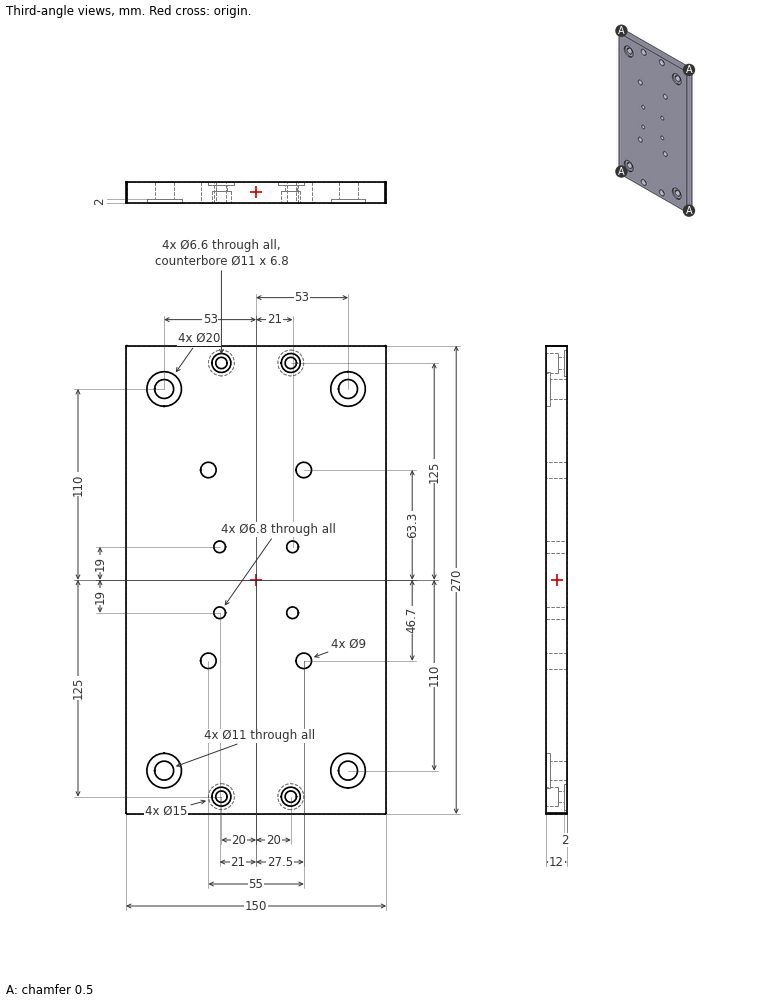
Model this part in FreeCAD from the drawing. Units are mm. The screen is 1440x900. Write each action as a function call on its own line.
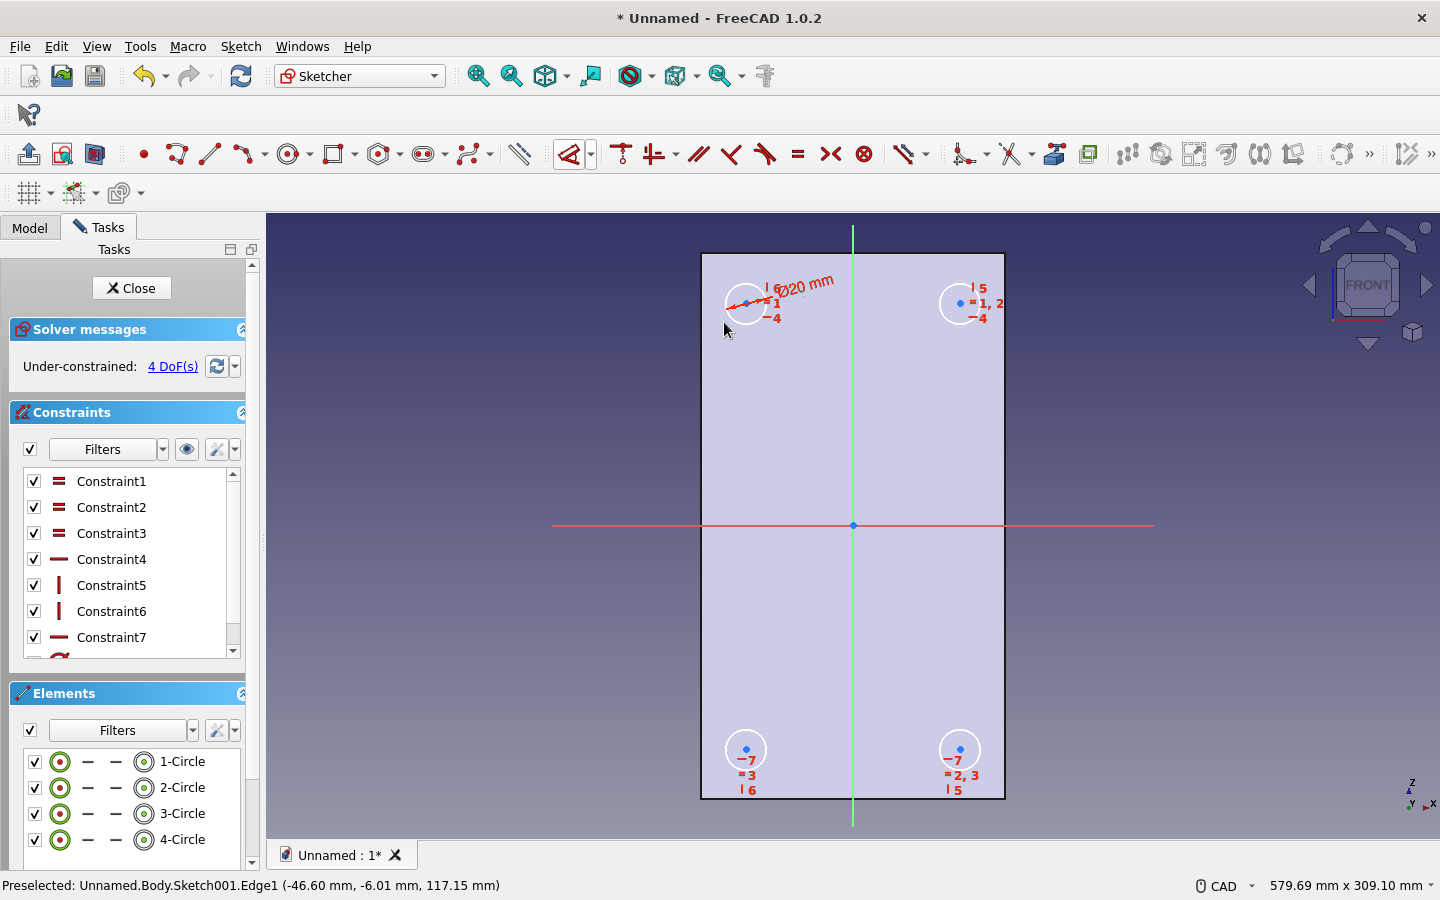
click(746, 304)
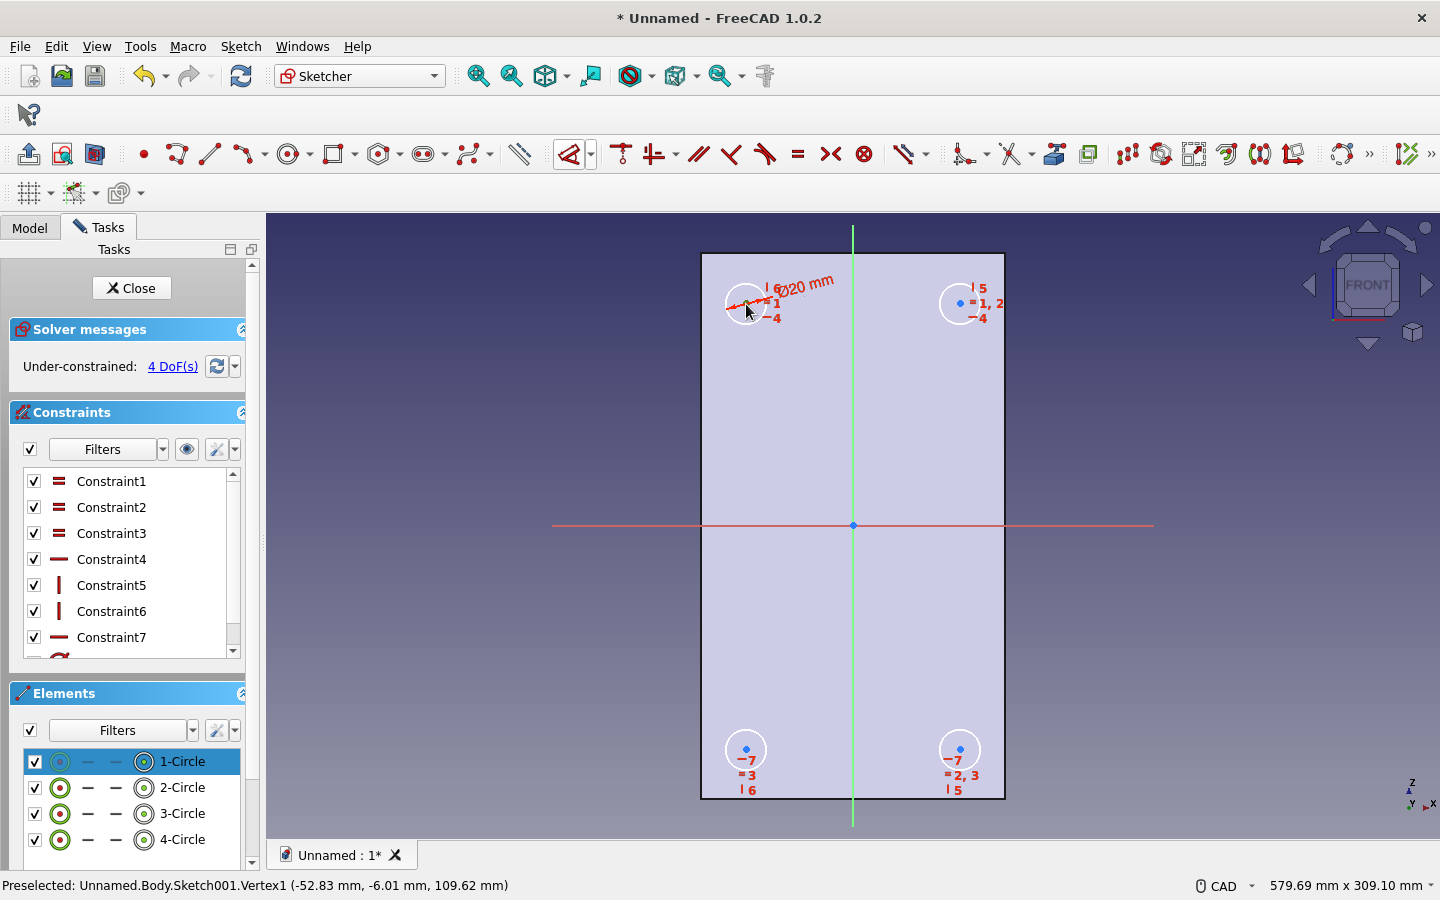
key(l)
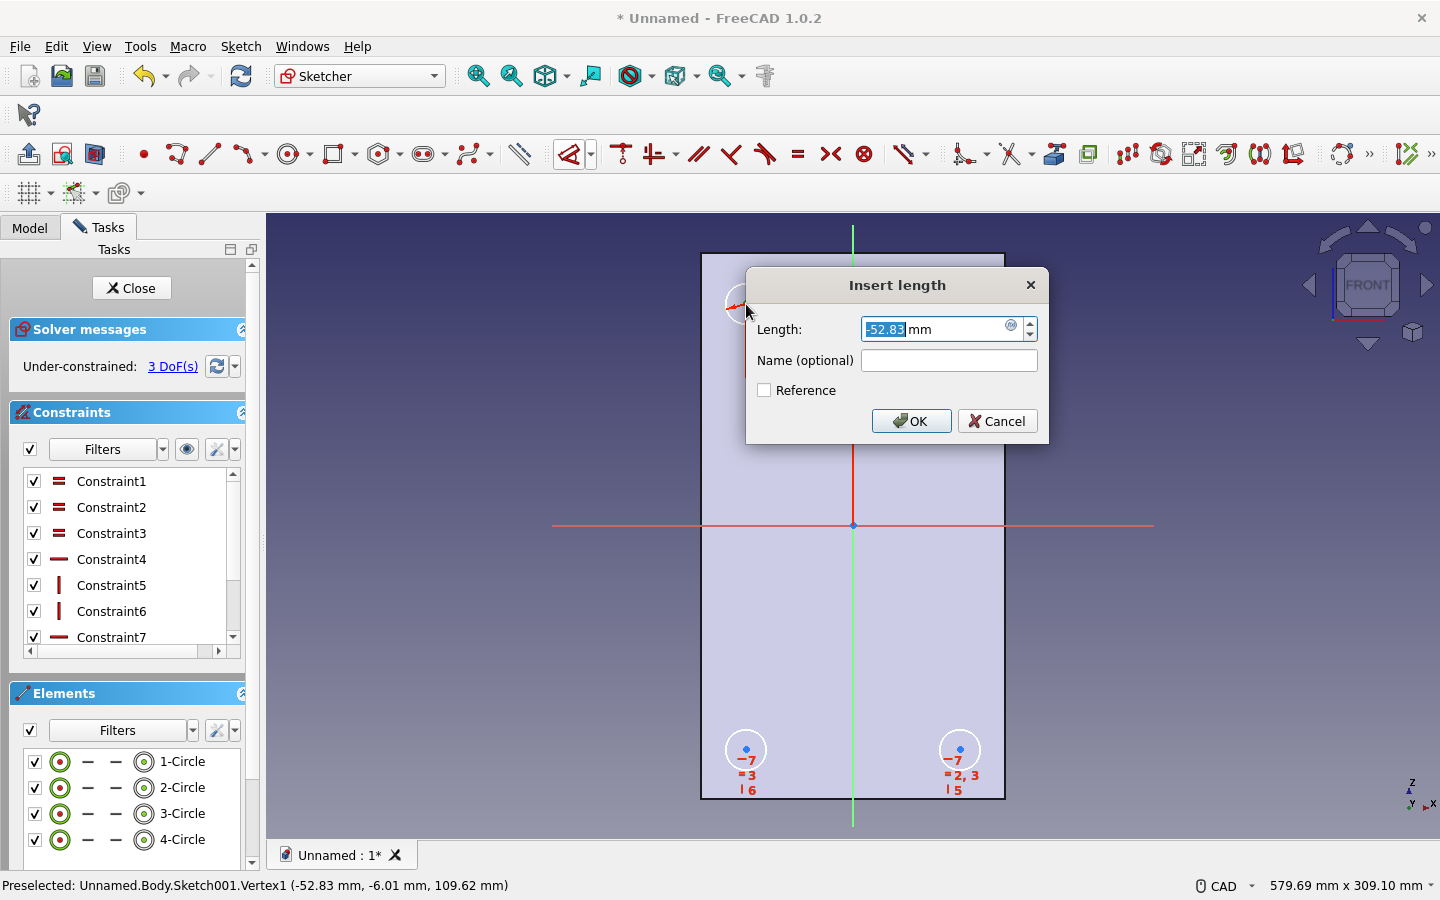
text(-53)
key(Return)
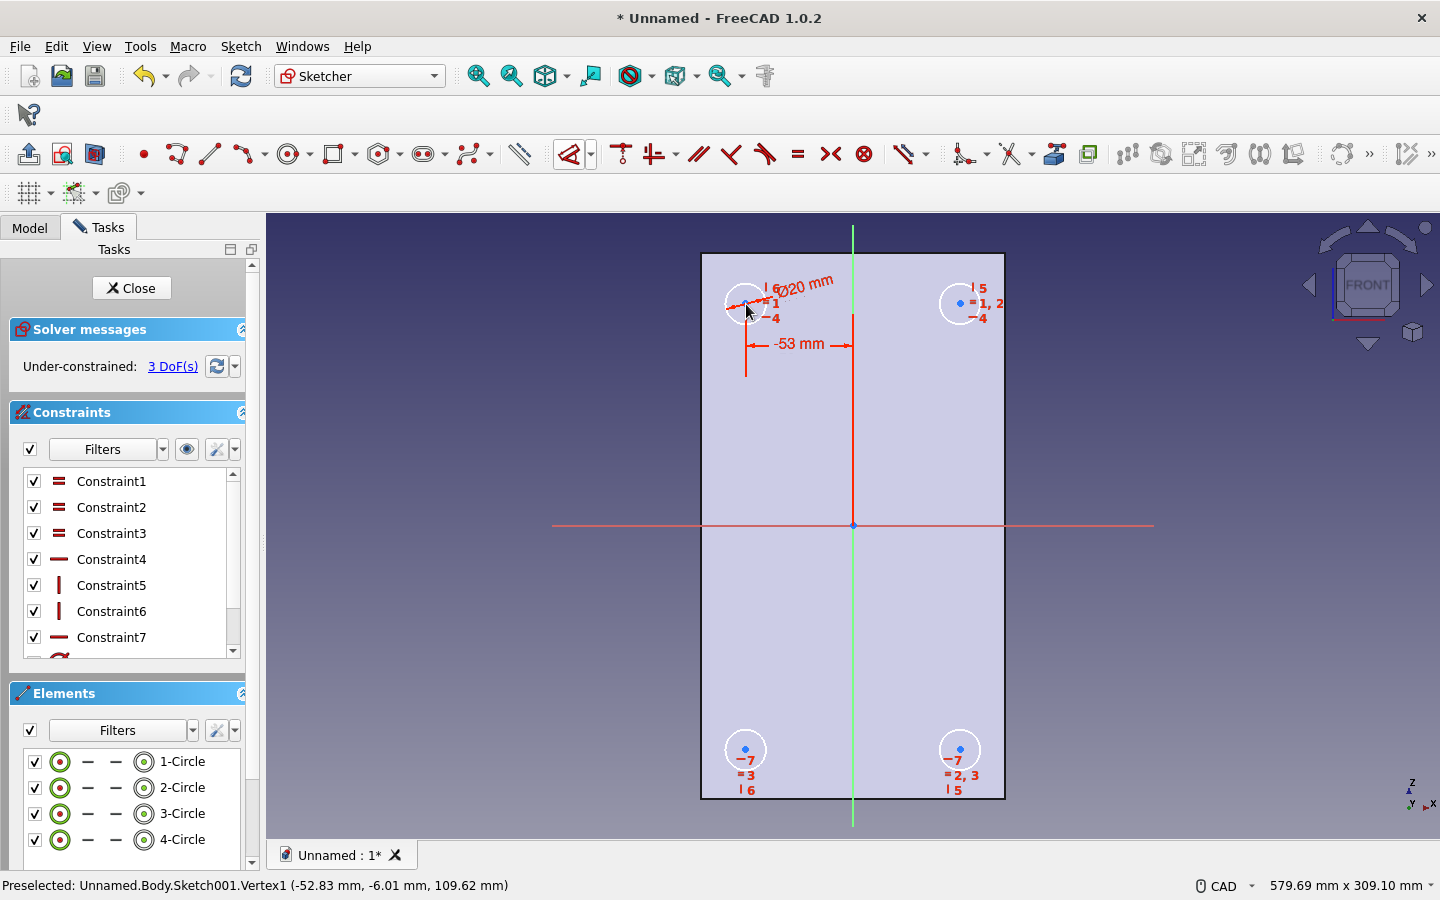
click(960, 304)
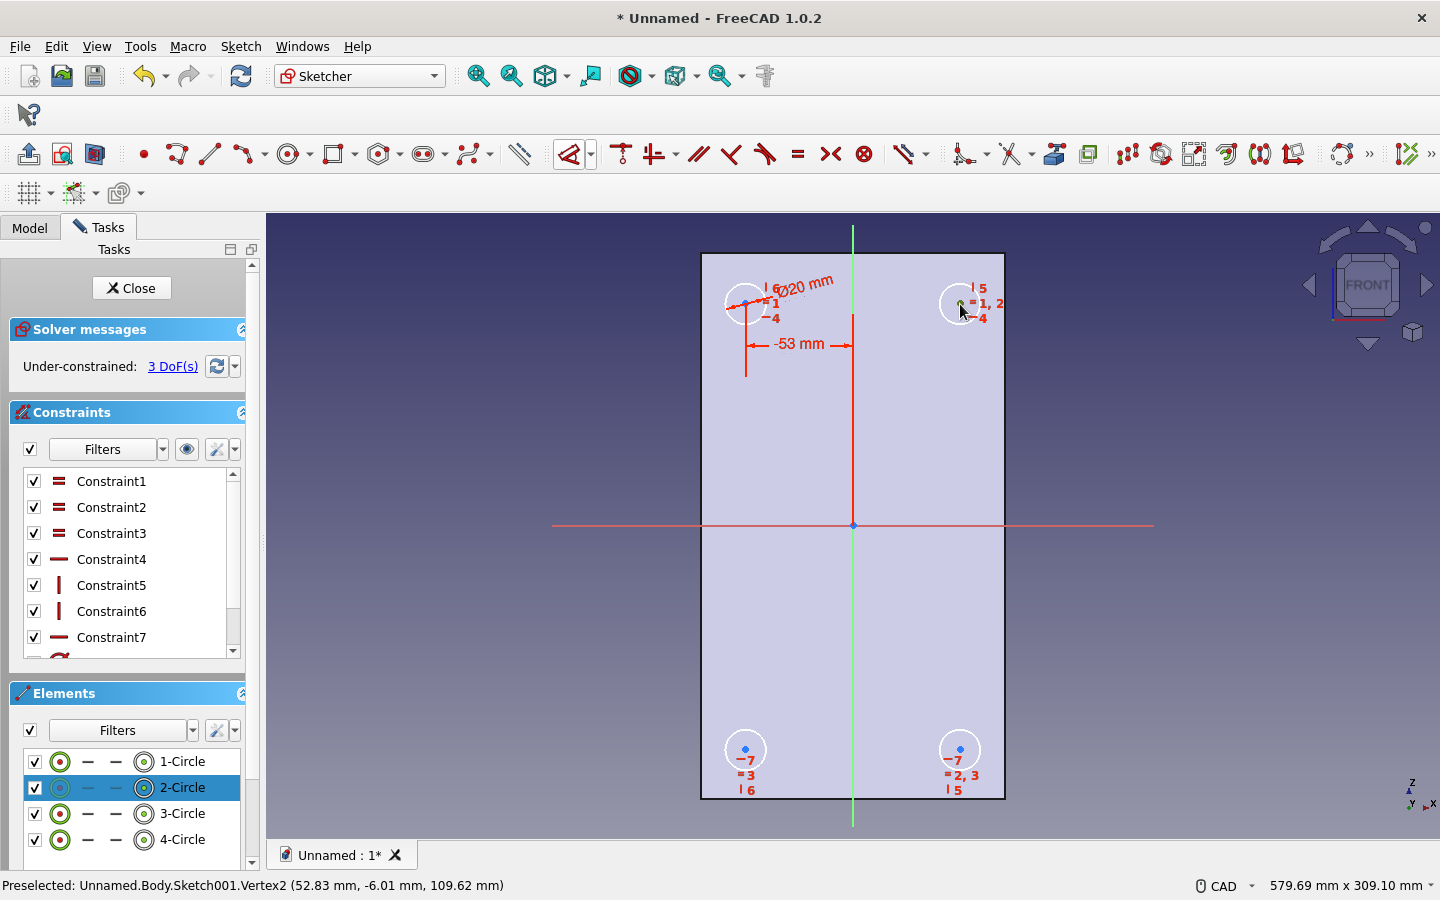
key(l)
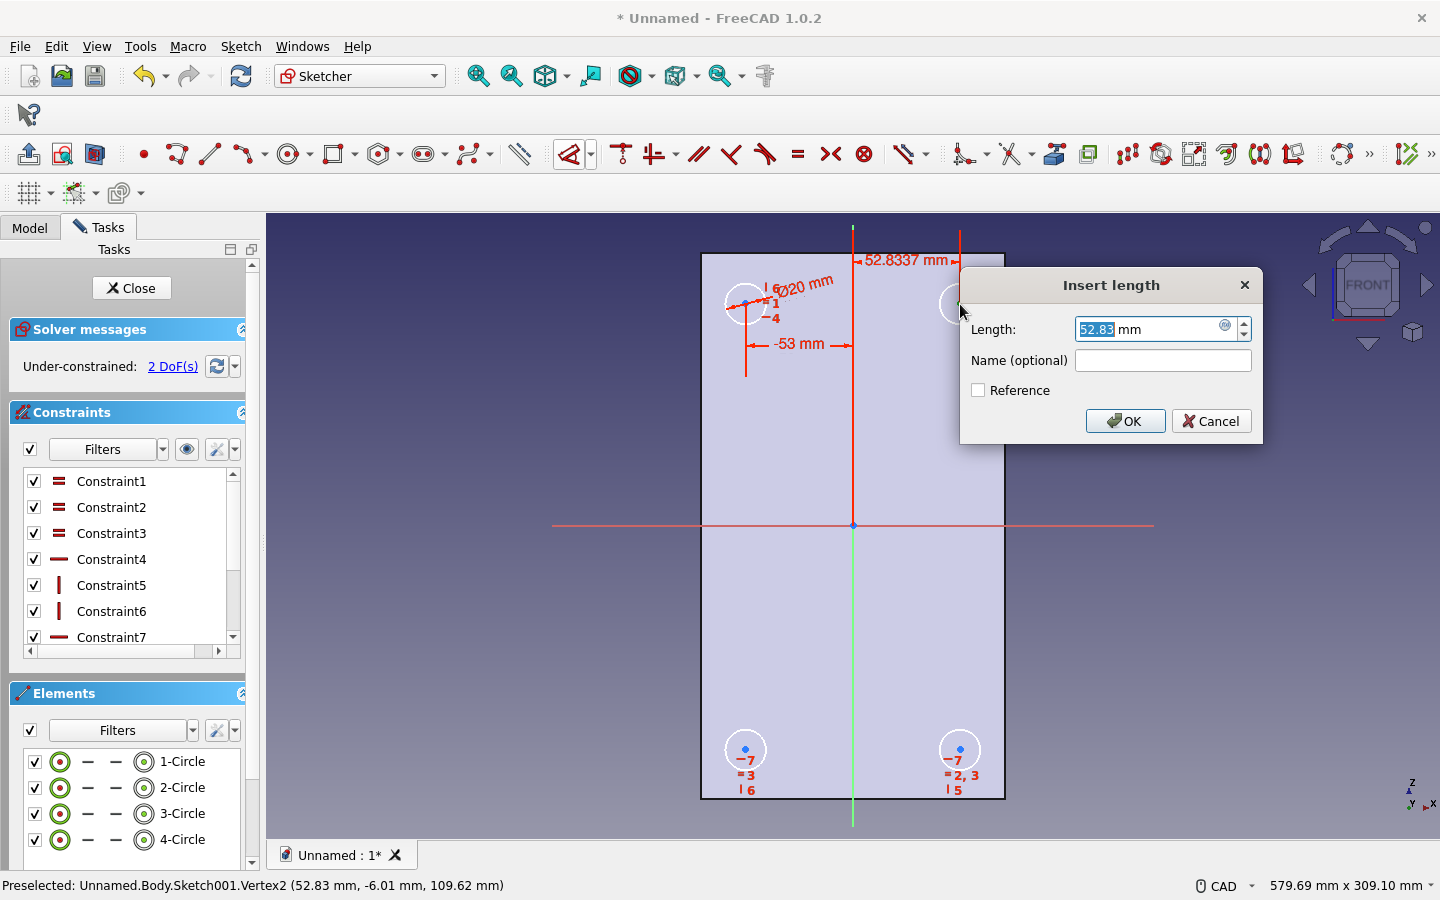
text(53)
key(Return)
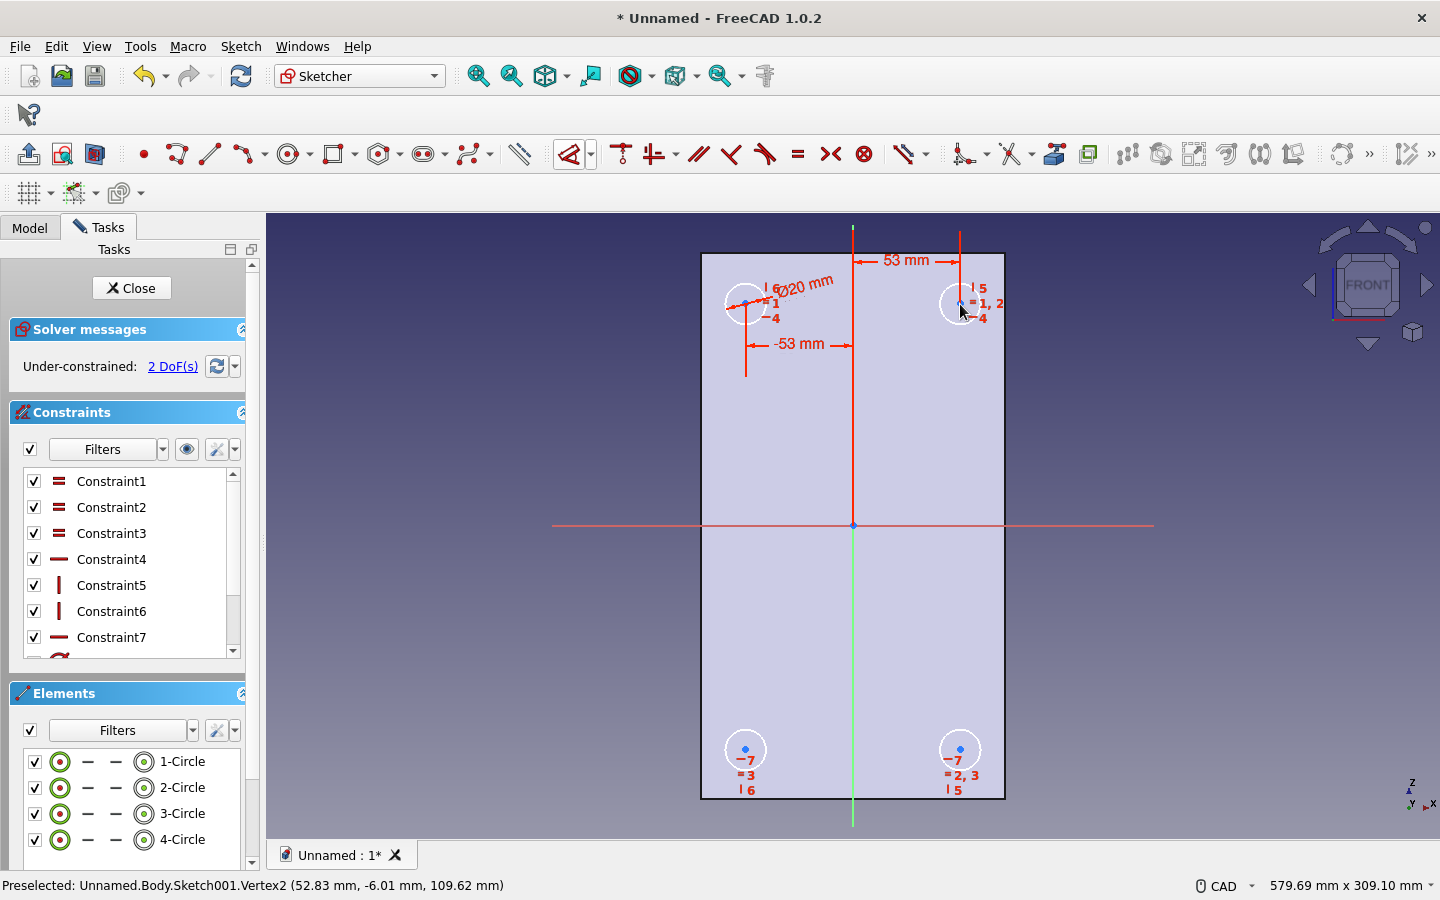
click(746, 304)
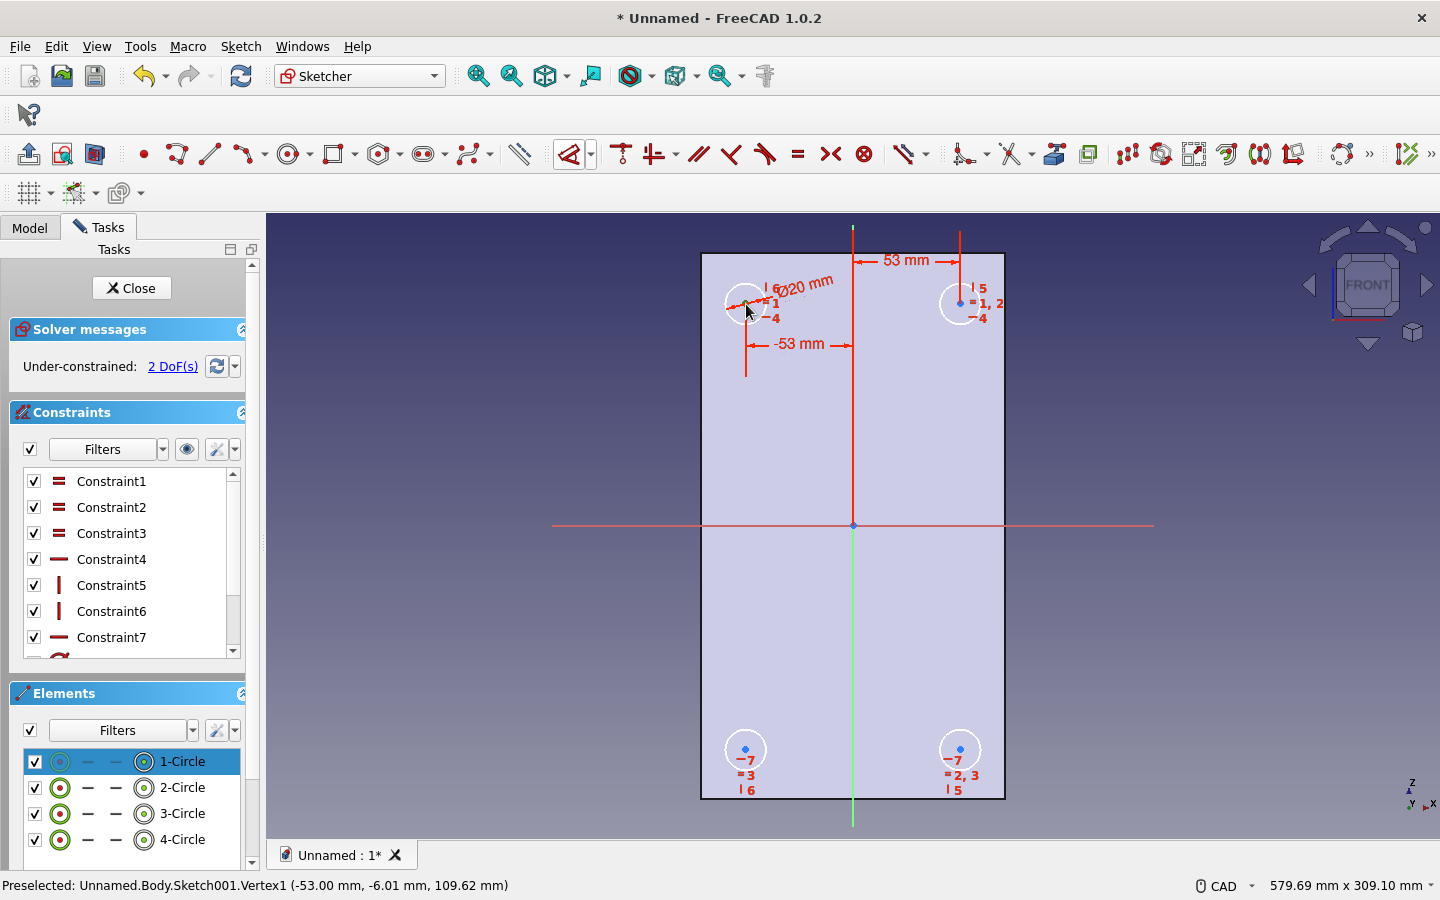
key(i)